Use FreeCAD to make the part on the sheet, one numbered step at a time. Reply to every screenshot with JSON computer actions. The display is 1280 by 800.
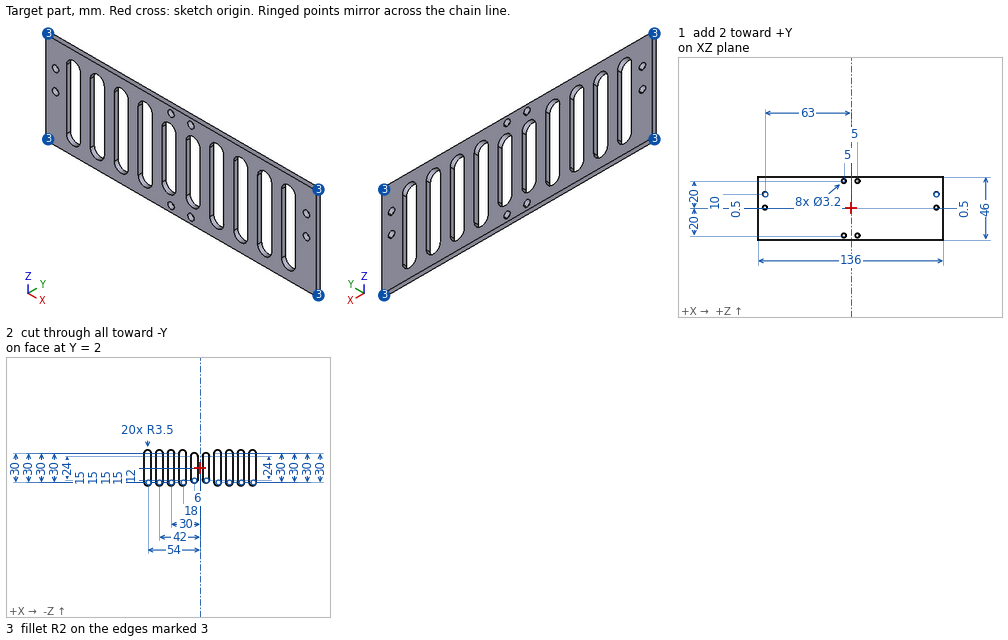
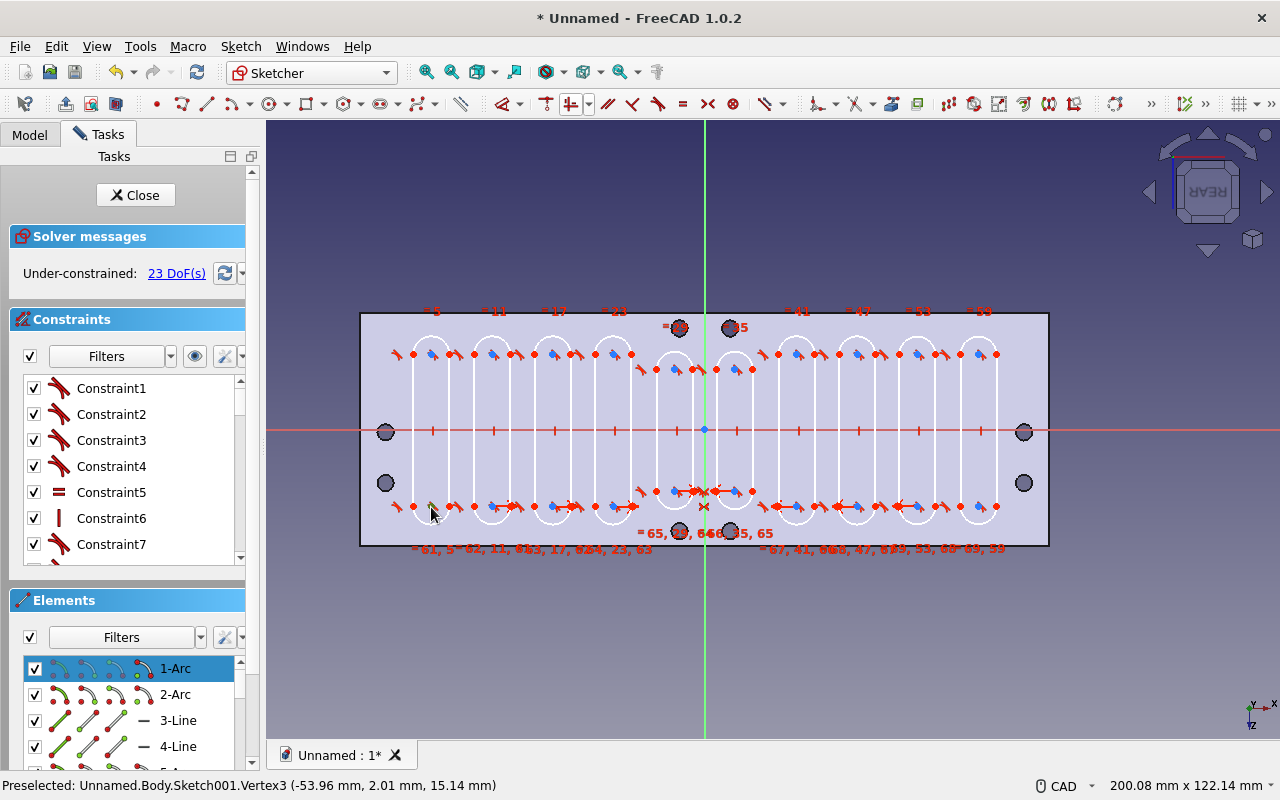
{"action": "left_click", "coordinate": [979, 506]}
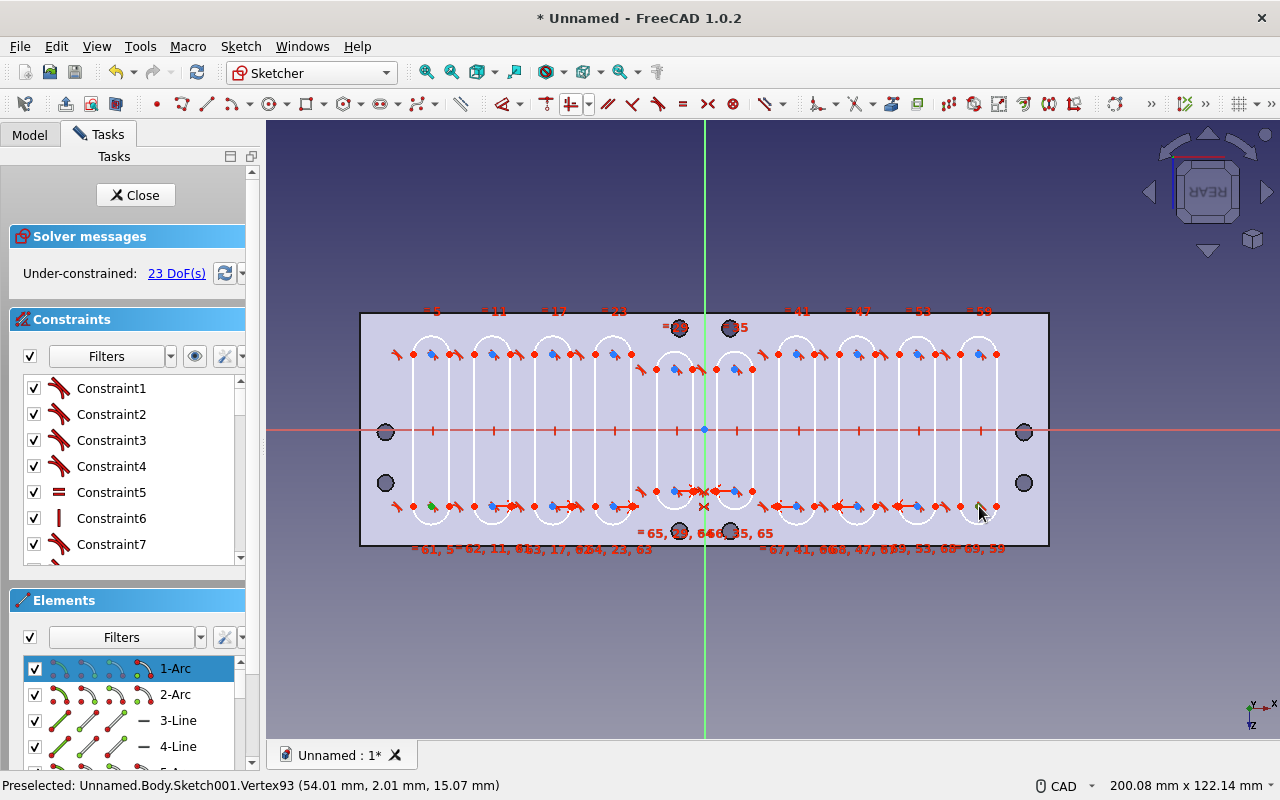
{"action": "left_click", "coordinate": [705, 671]}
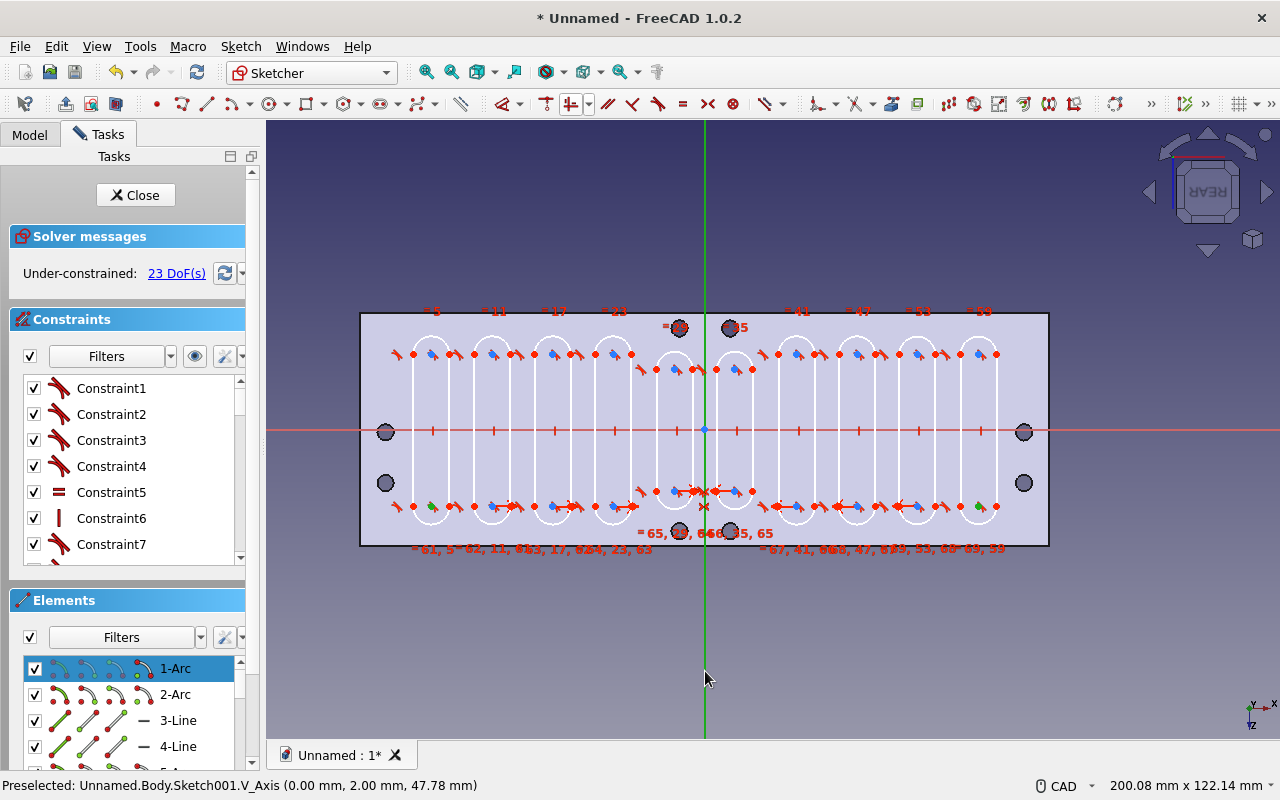
{"action": "left_click", "coordinate": [708, 104]}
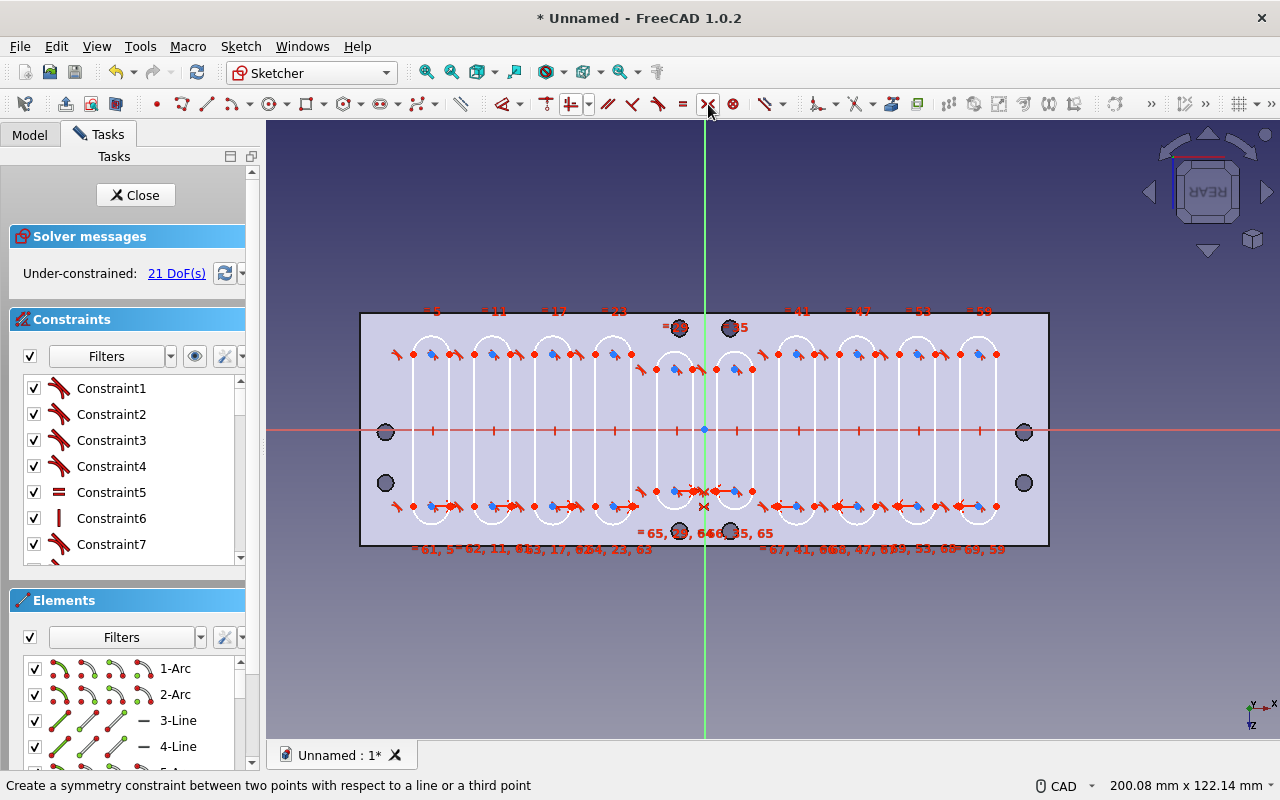
{"action": "left_click", "coordinate": [502, 104]}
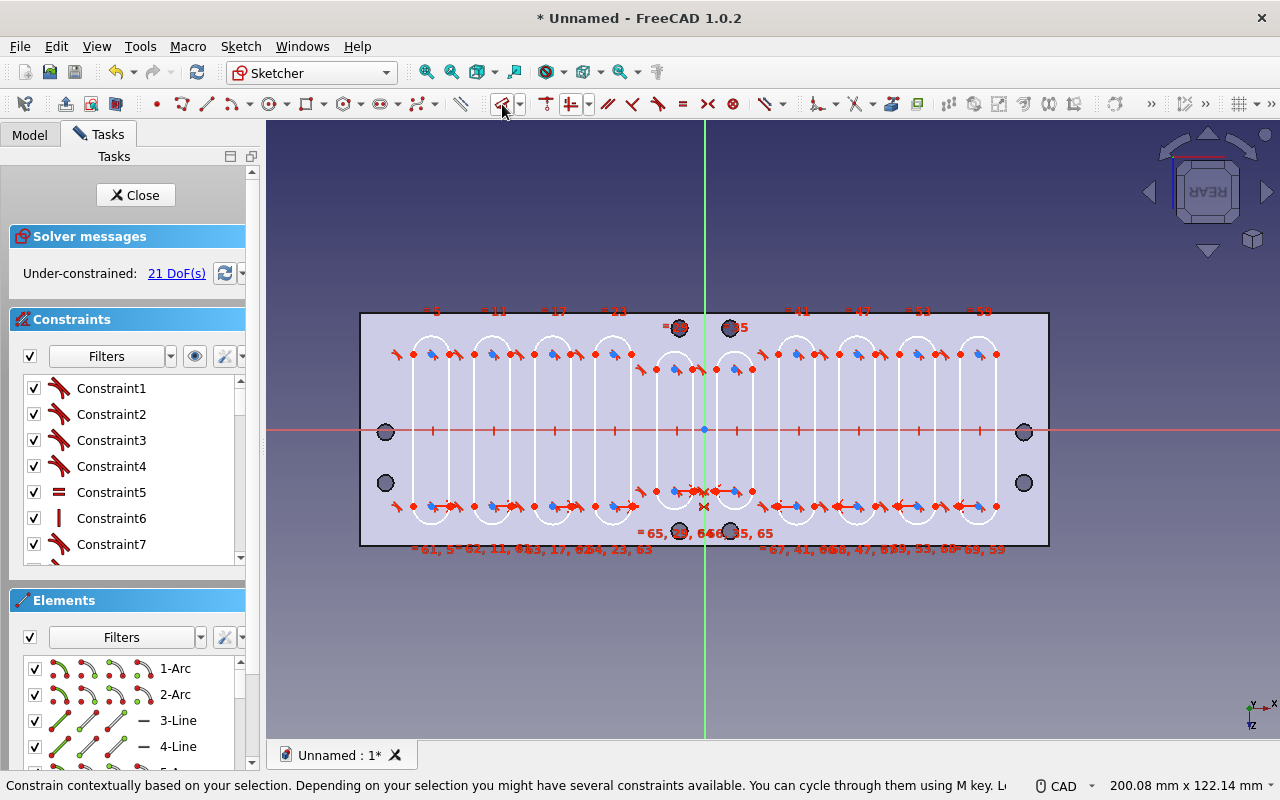
{"action": "scroll", "coordinate": [421, 521], "scroll_direction": "up", "scroll_amount": 5}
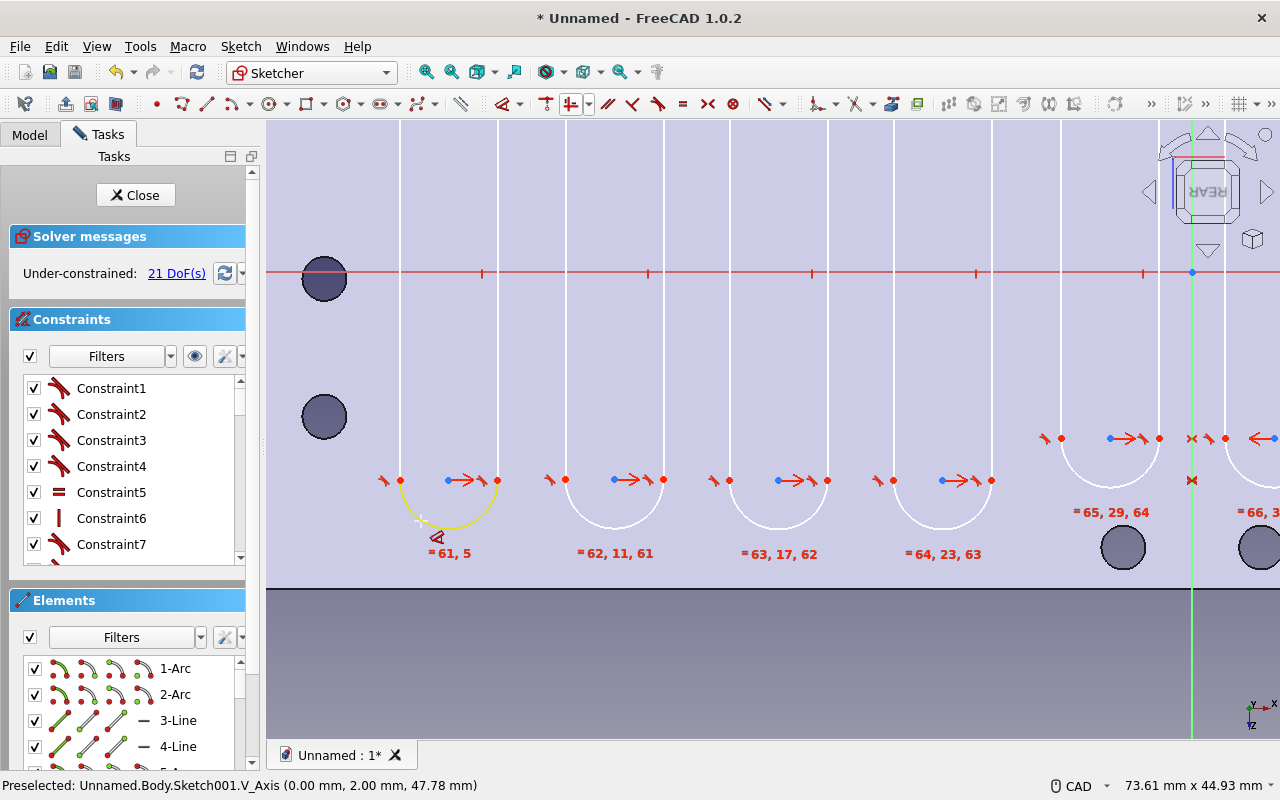
{"action": "left_click", "coordinate": [420, 520]}
{"action": "left_click", "coordinate": [401, 546]}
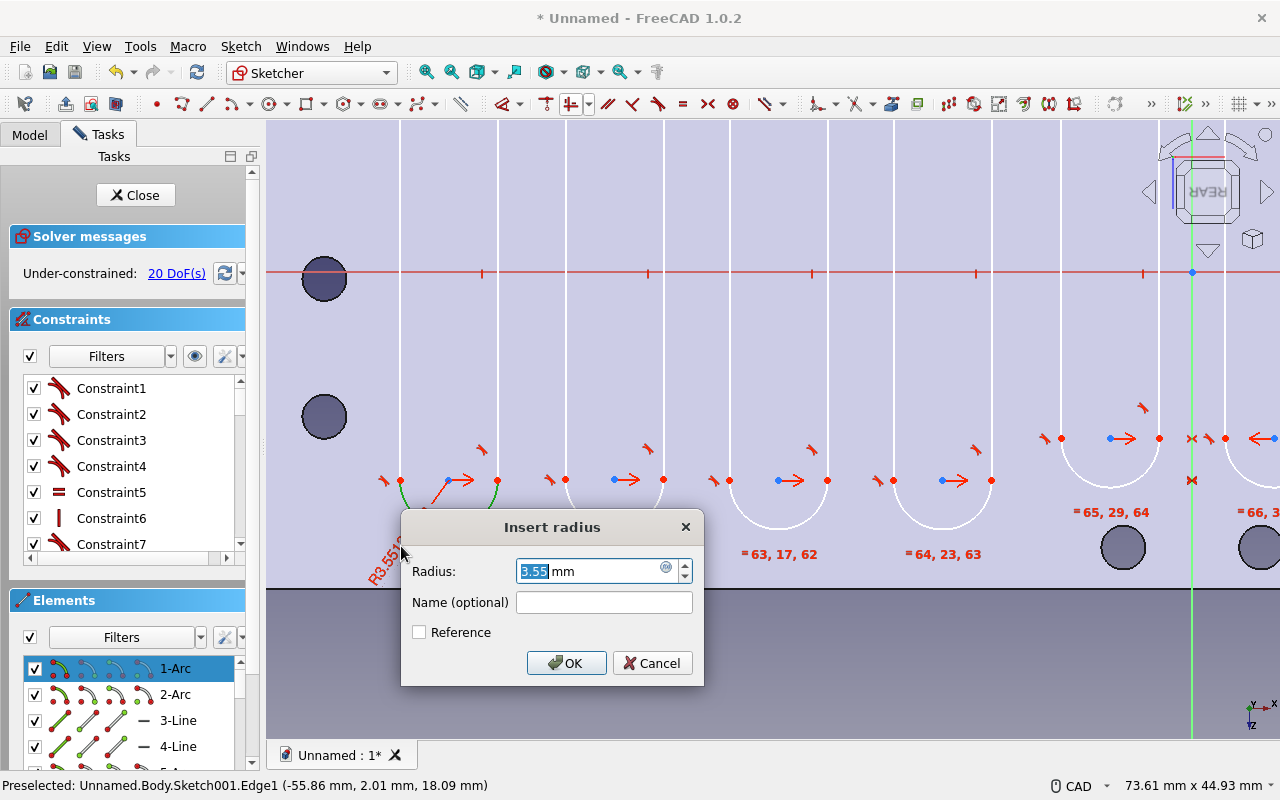
{"action": "type", "text": "3.5"}
{"action": "key", "text": "Return"}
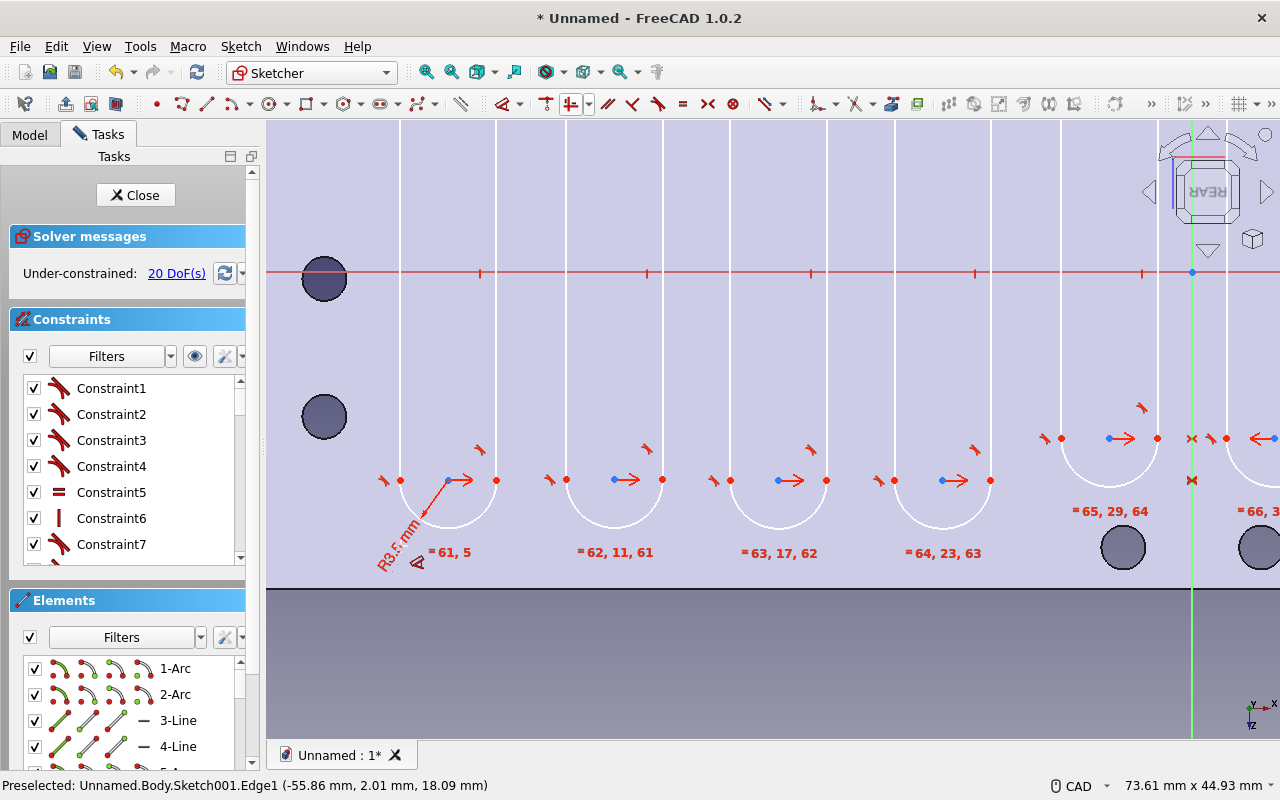
{"action": "left_click", "coordinate": [400, 356]}
{"action": "left_click", "coordinate": [366, 314]}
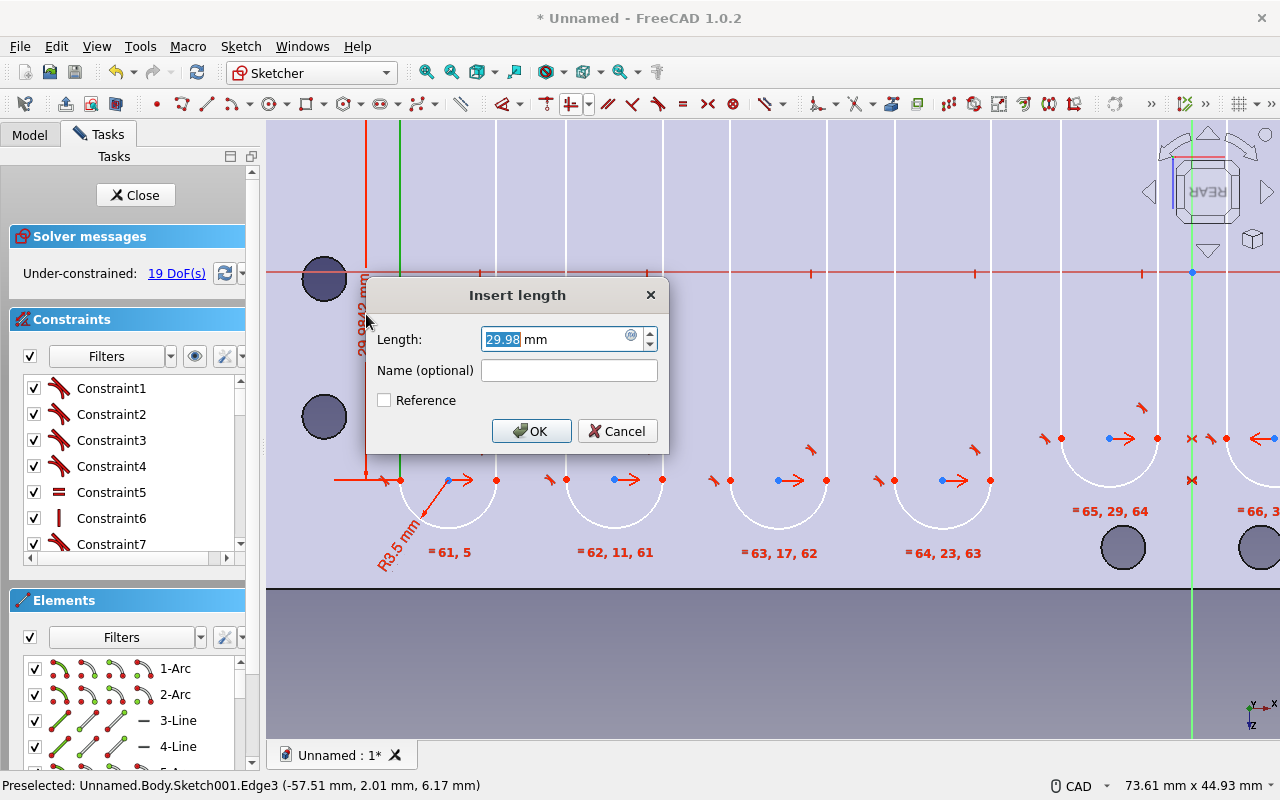
{"action": "type", "text": "30"}
{"action": "key", "text": "Return"}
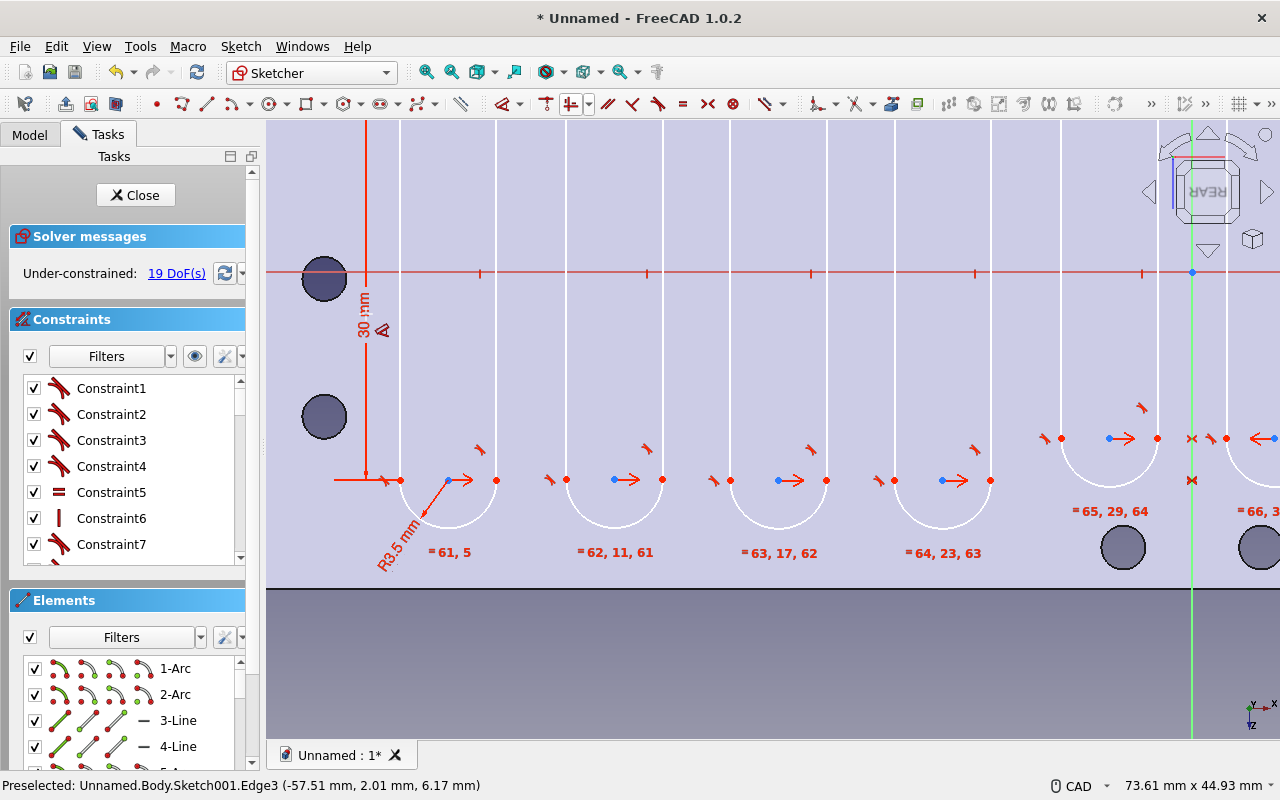
{"action": "left_click", "coordinate": [566, 356]}
{"action": "left_click", "coordinate": [532, 314]}